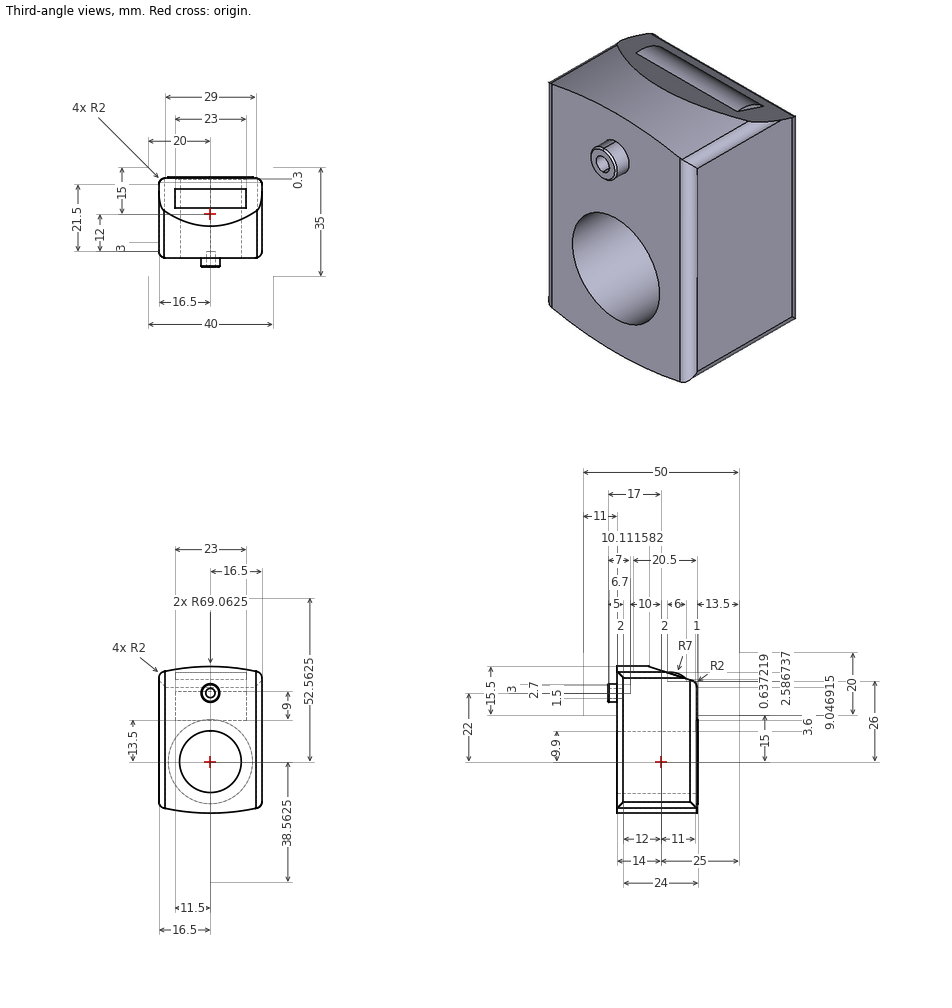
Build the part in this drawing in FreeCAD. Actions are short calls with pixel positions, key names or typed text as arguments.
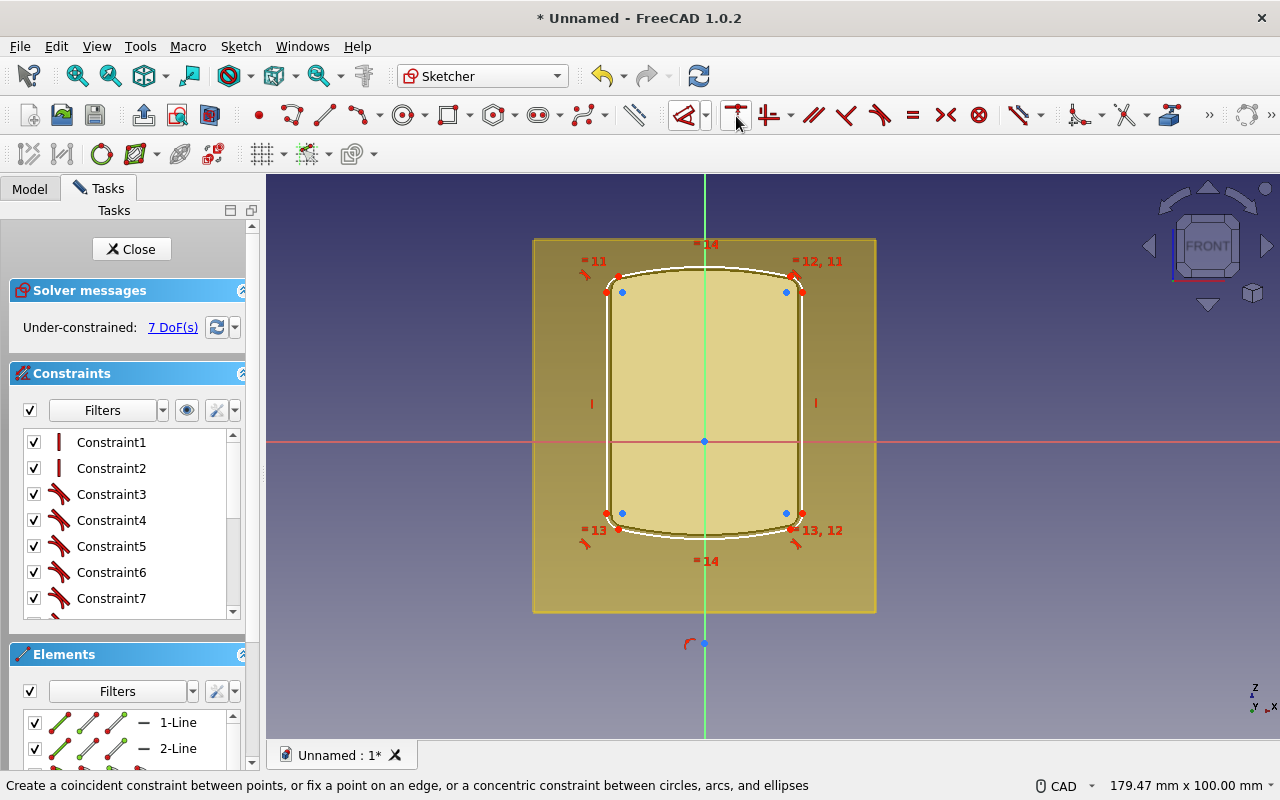
scroll(705, 292, up, 2)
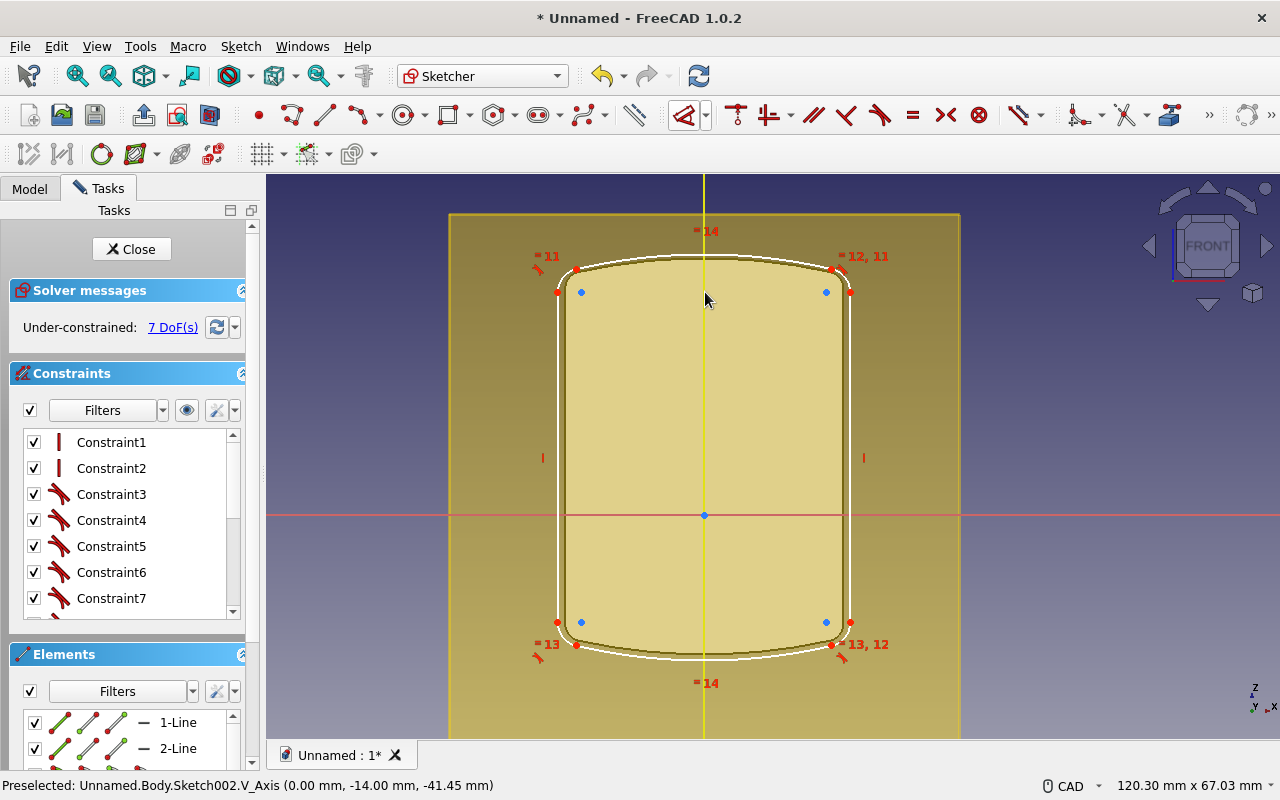
scroll(705, 620, down, 2)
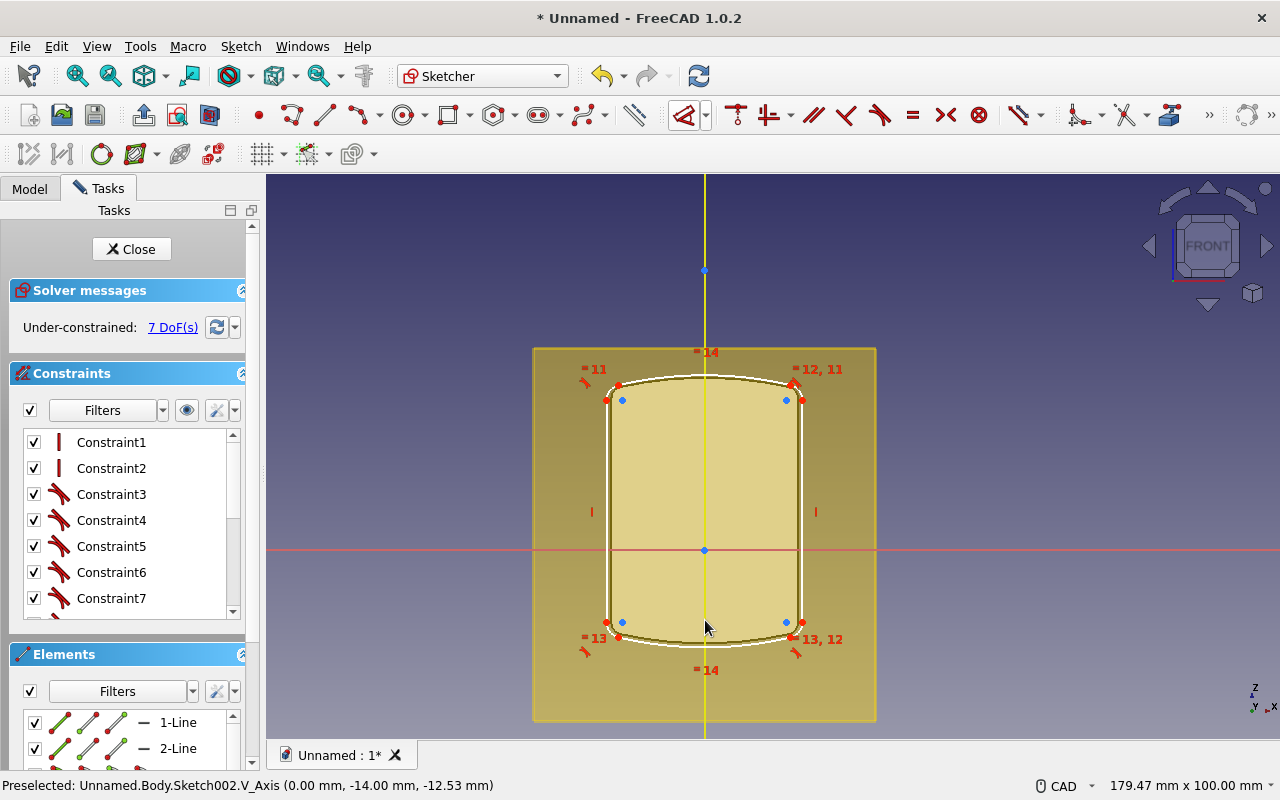
click(705, 270)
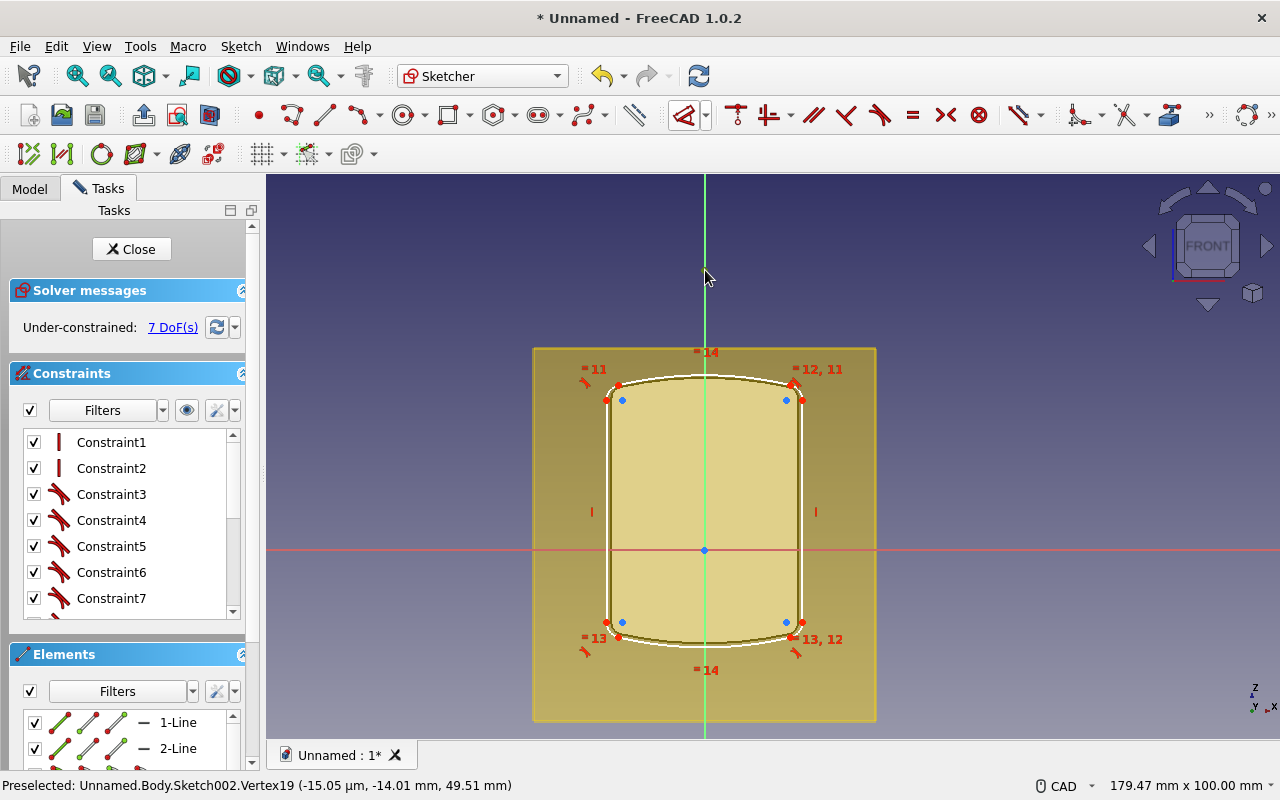
click(705, 602)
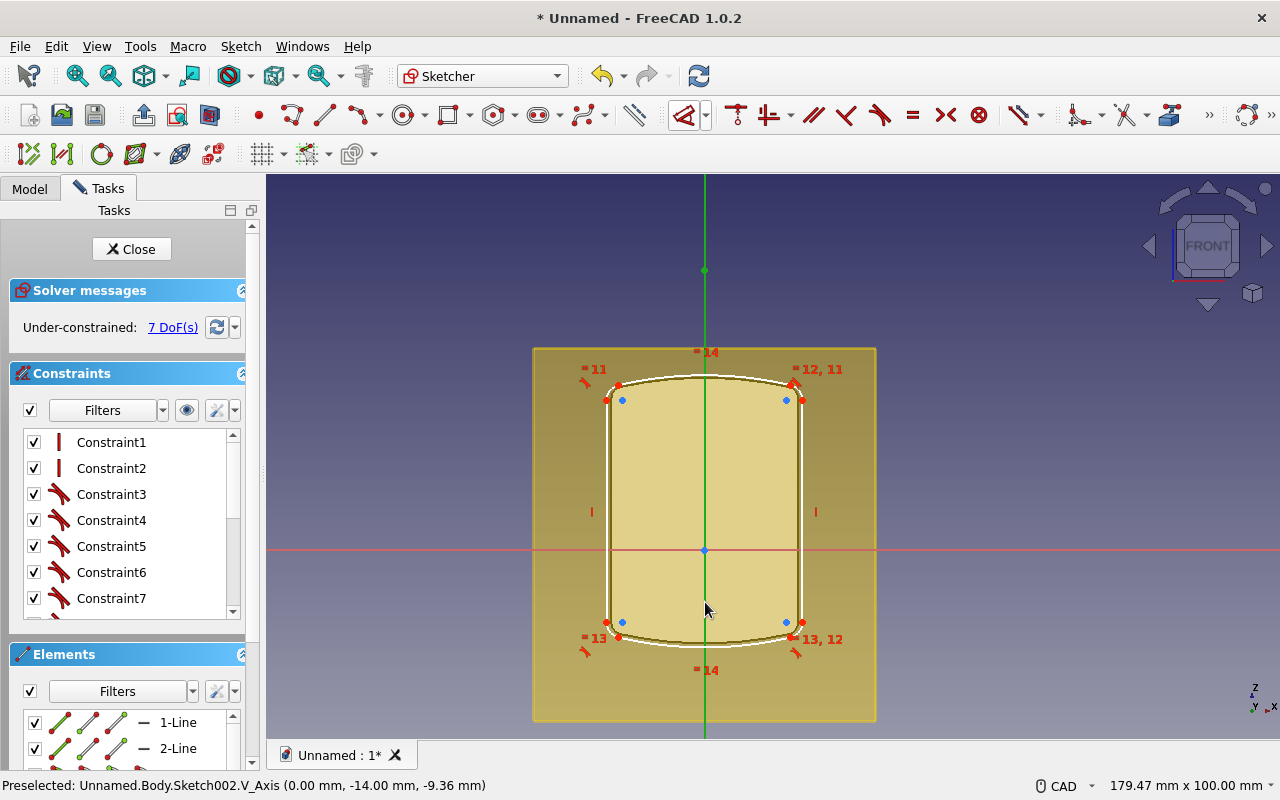
click(736, 116)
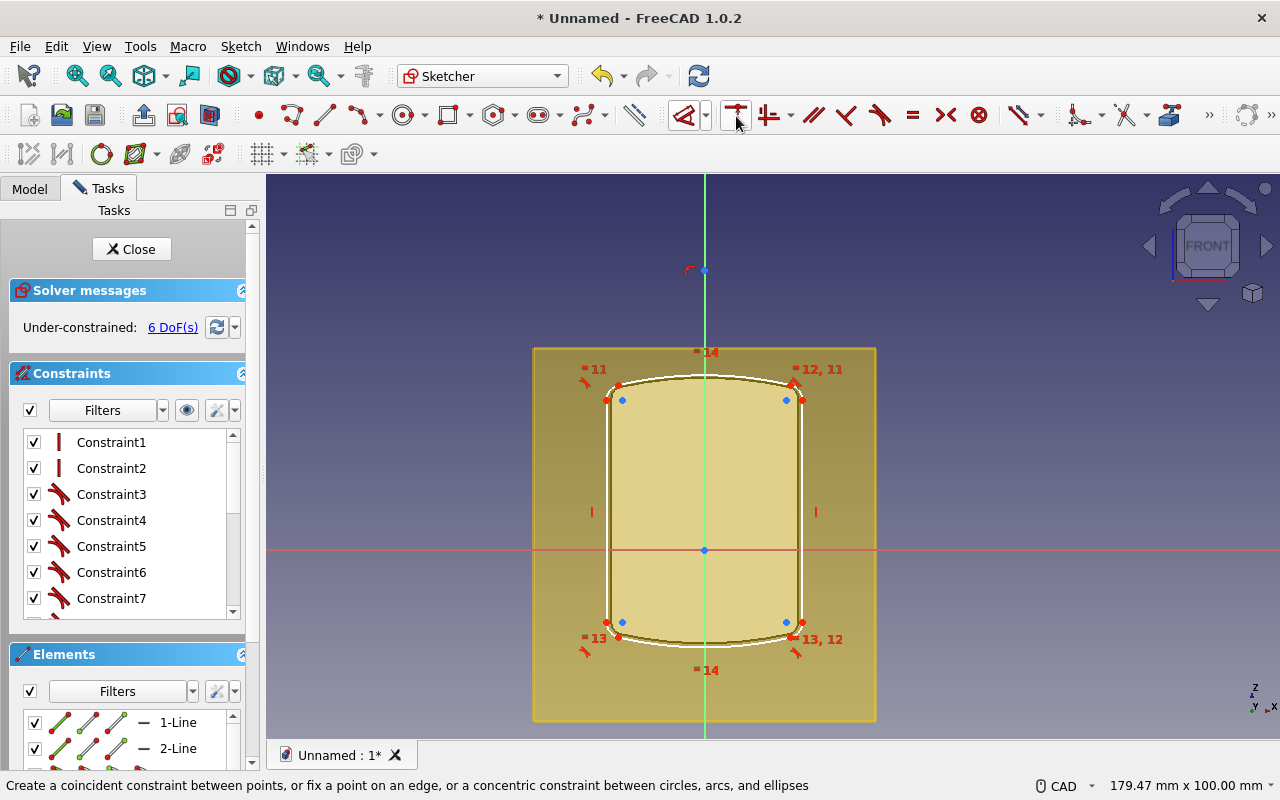
scroll(610, 391, up, 7)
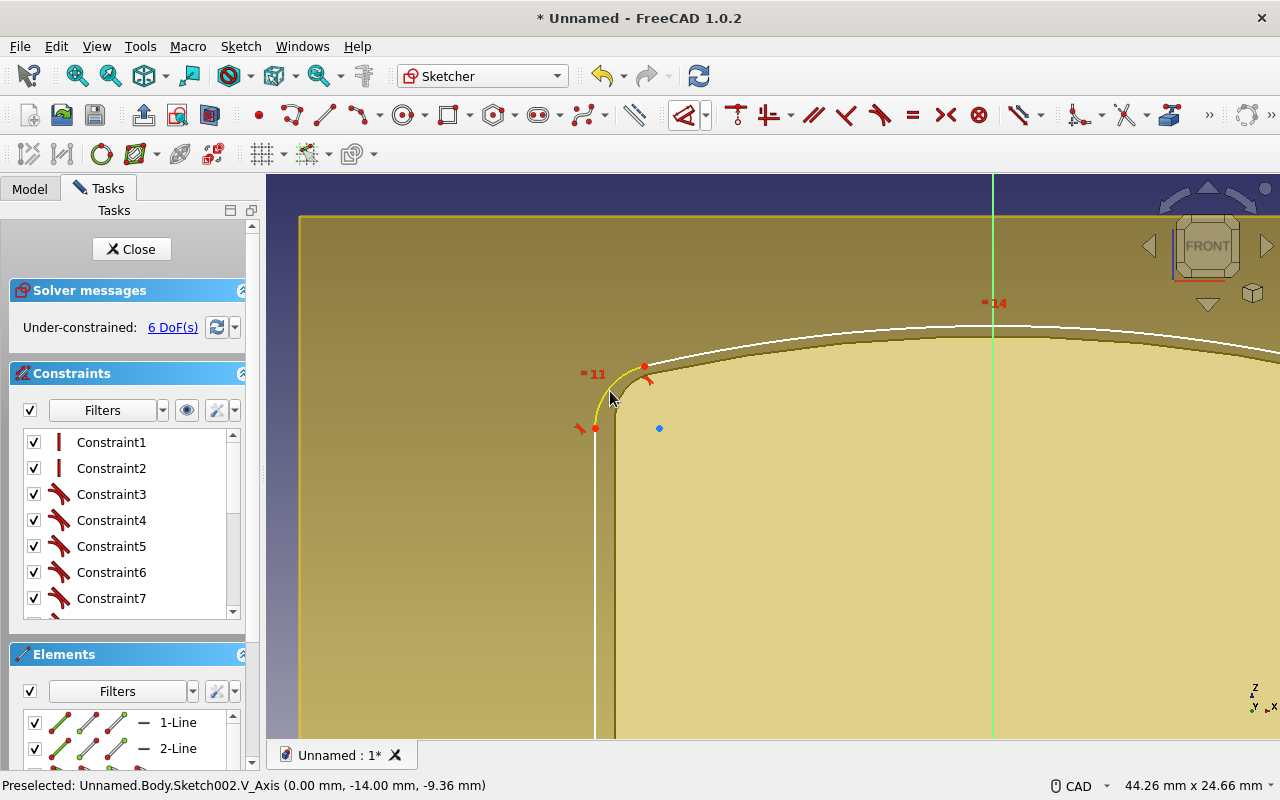
click(609, 389)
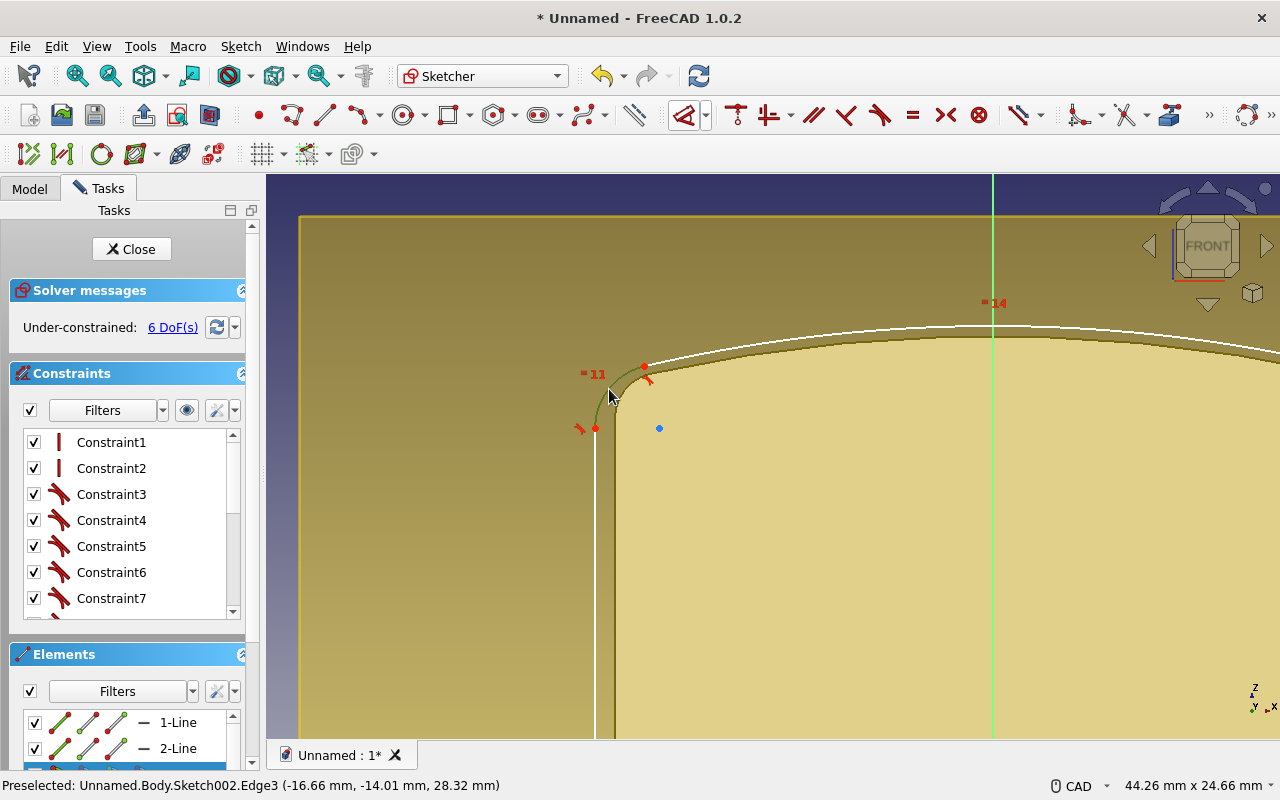
key(k)
key(r)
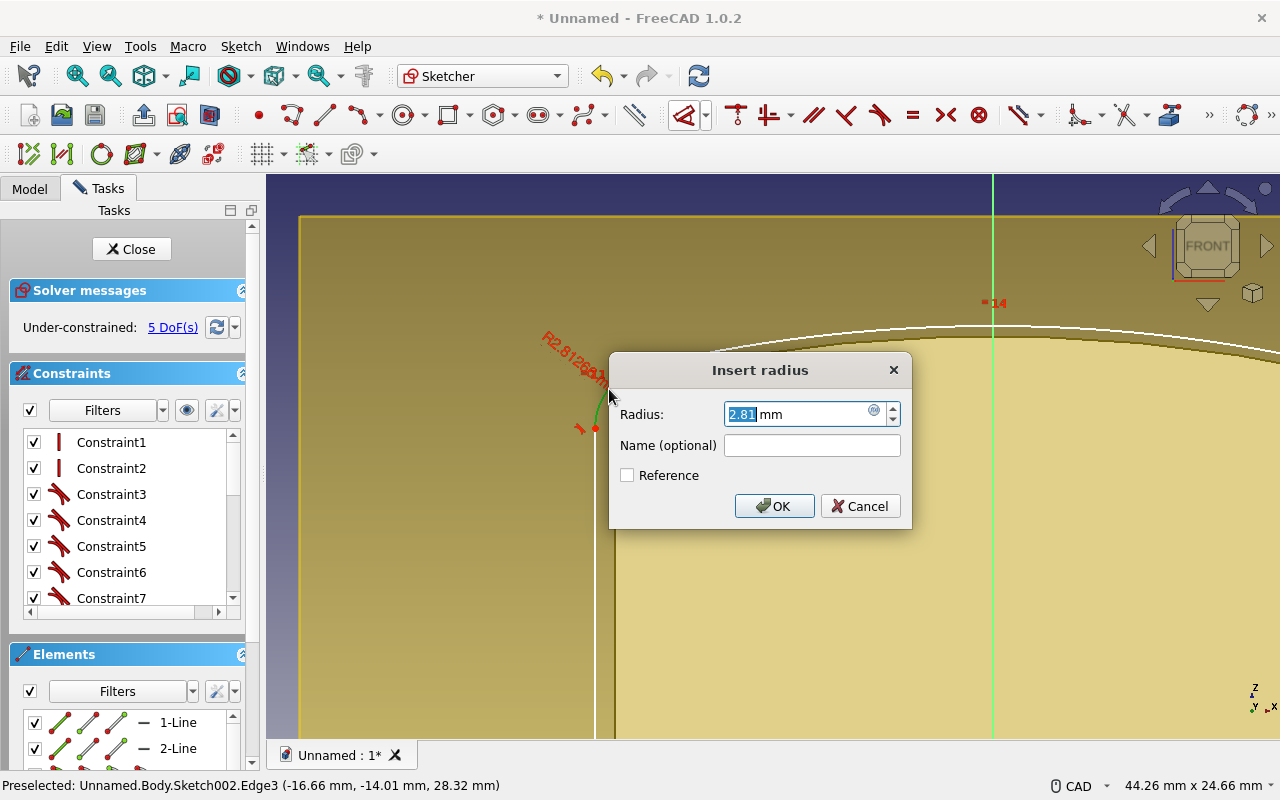
text(2)
key(Return)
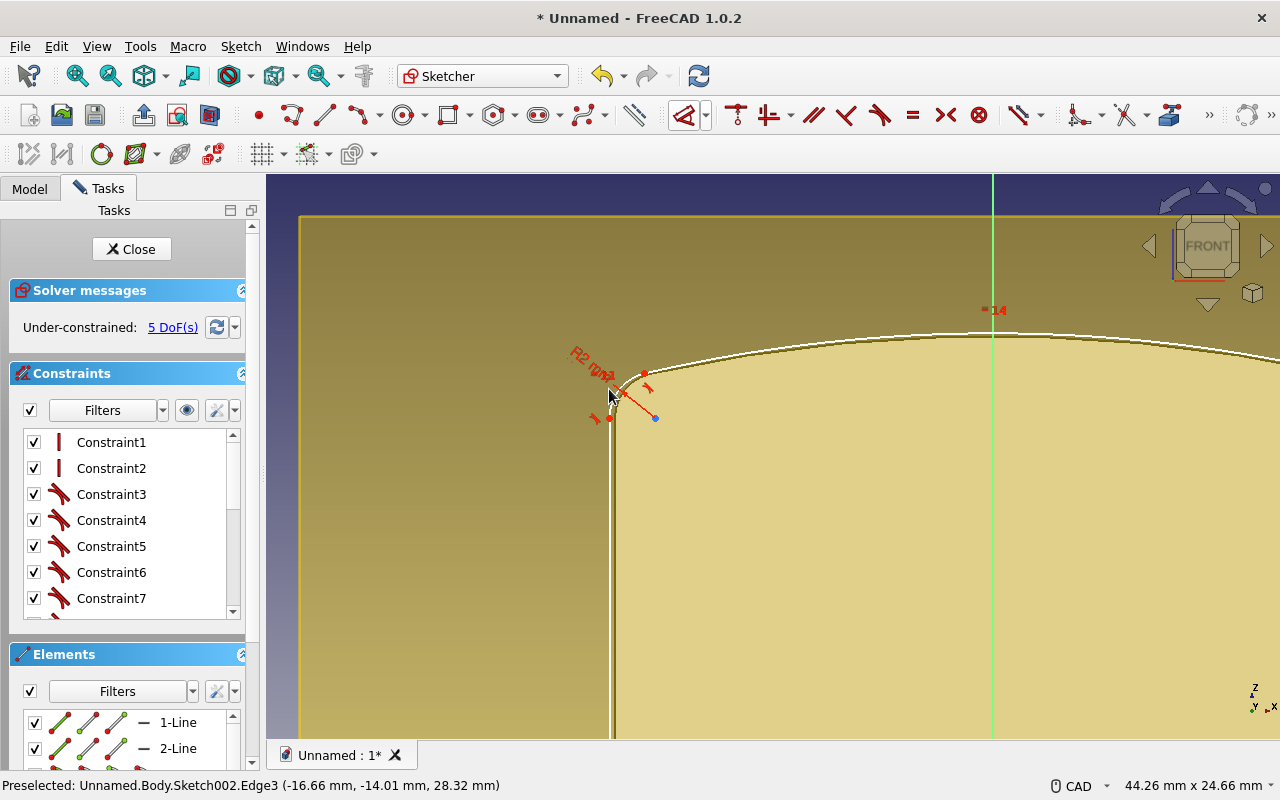
click(852, 340)